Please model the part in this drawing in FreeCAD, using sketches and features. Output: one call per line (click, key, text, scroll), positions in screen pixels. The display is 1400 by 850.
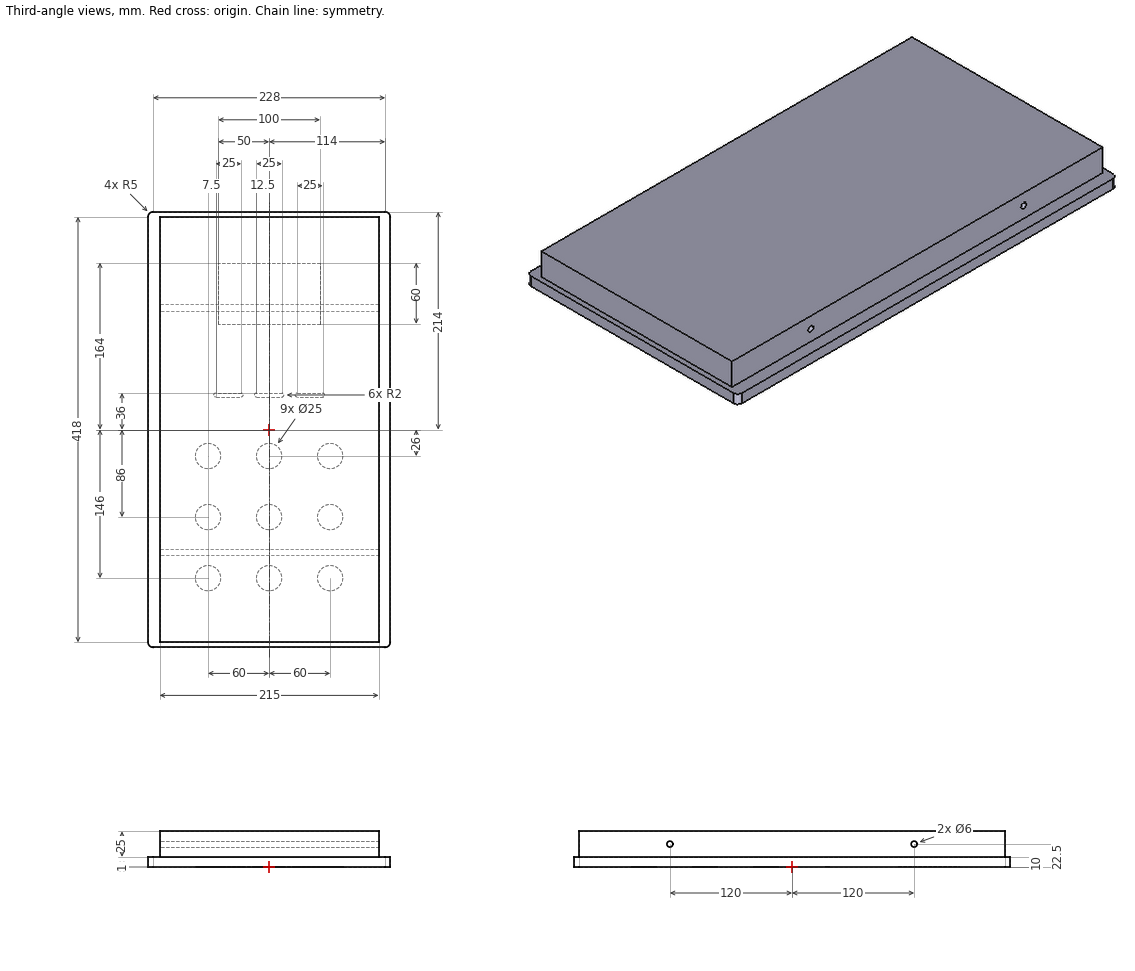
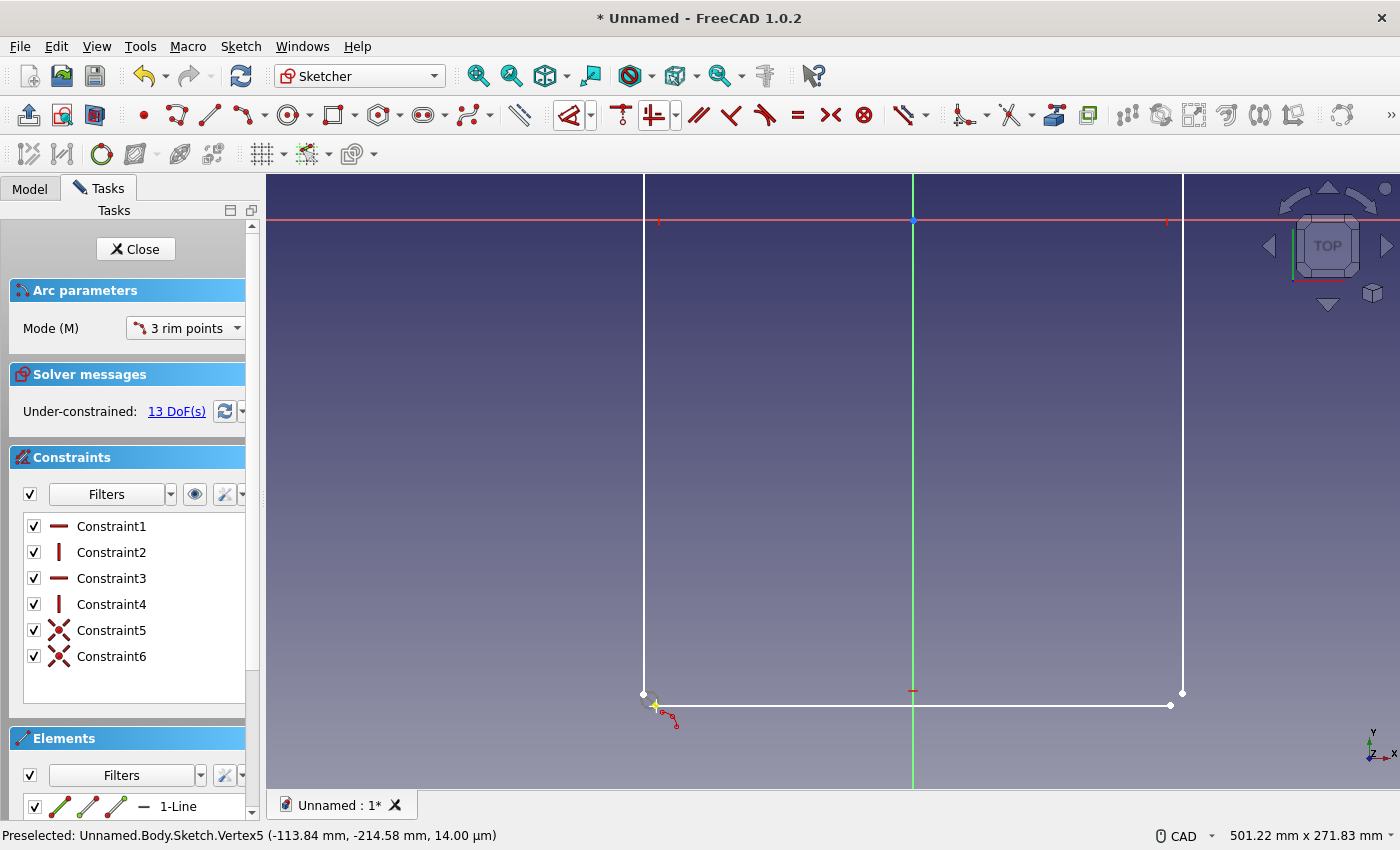
scroll(648, 701, up, 8)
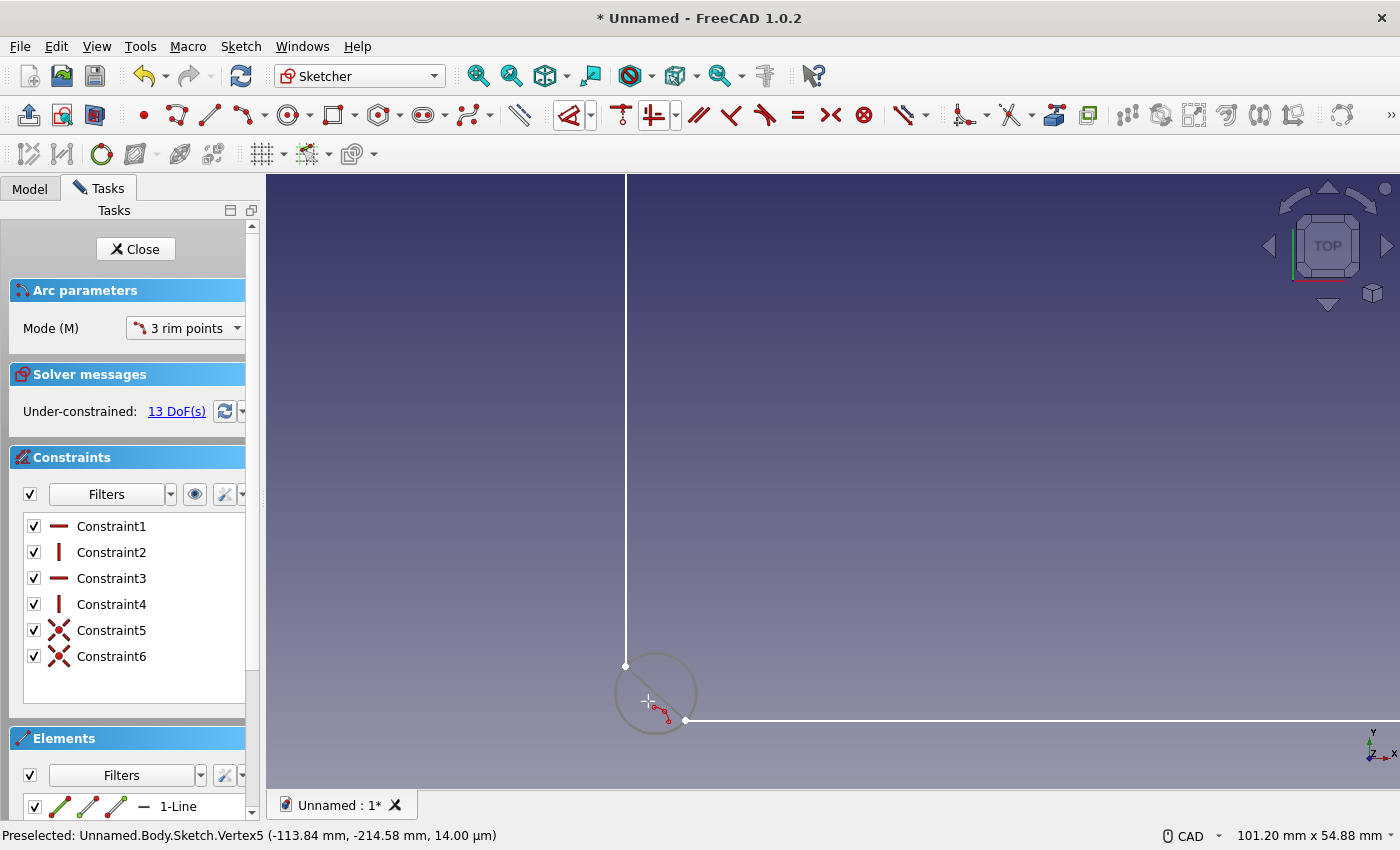
click(644, 698)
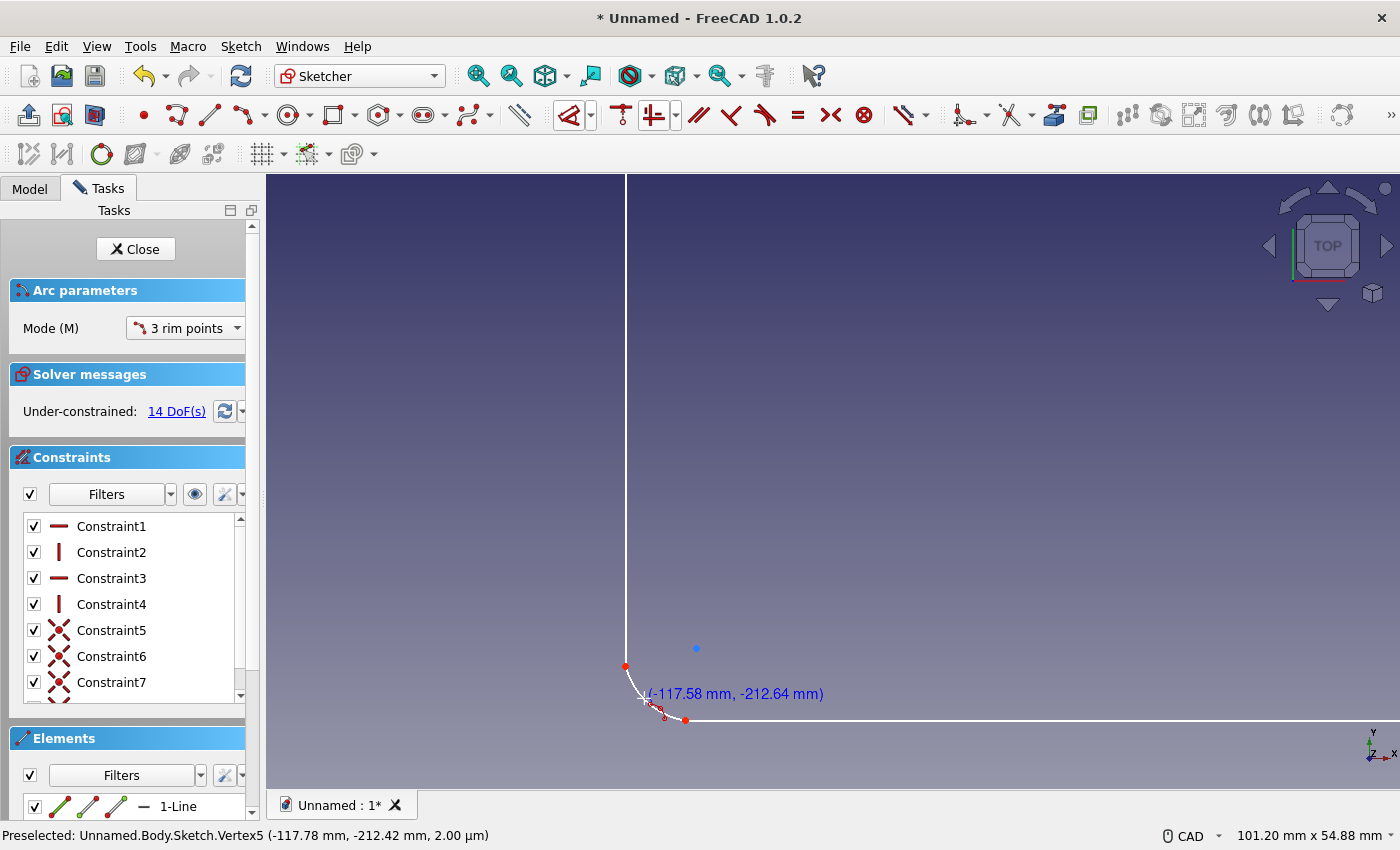
scroll(645, 698, down, 12)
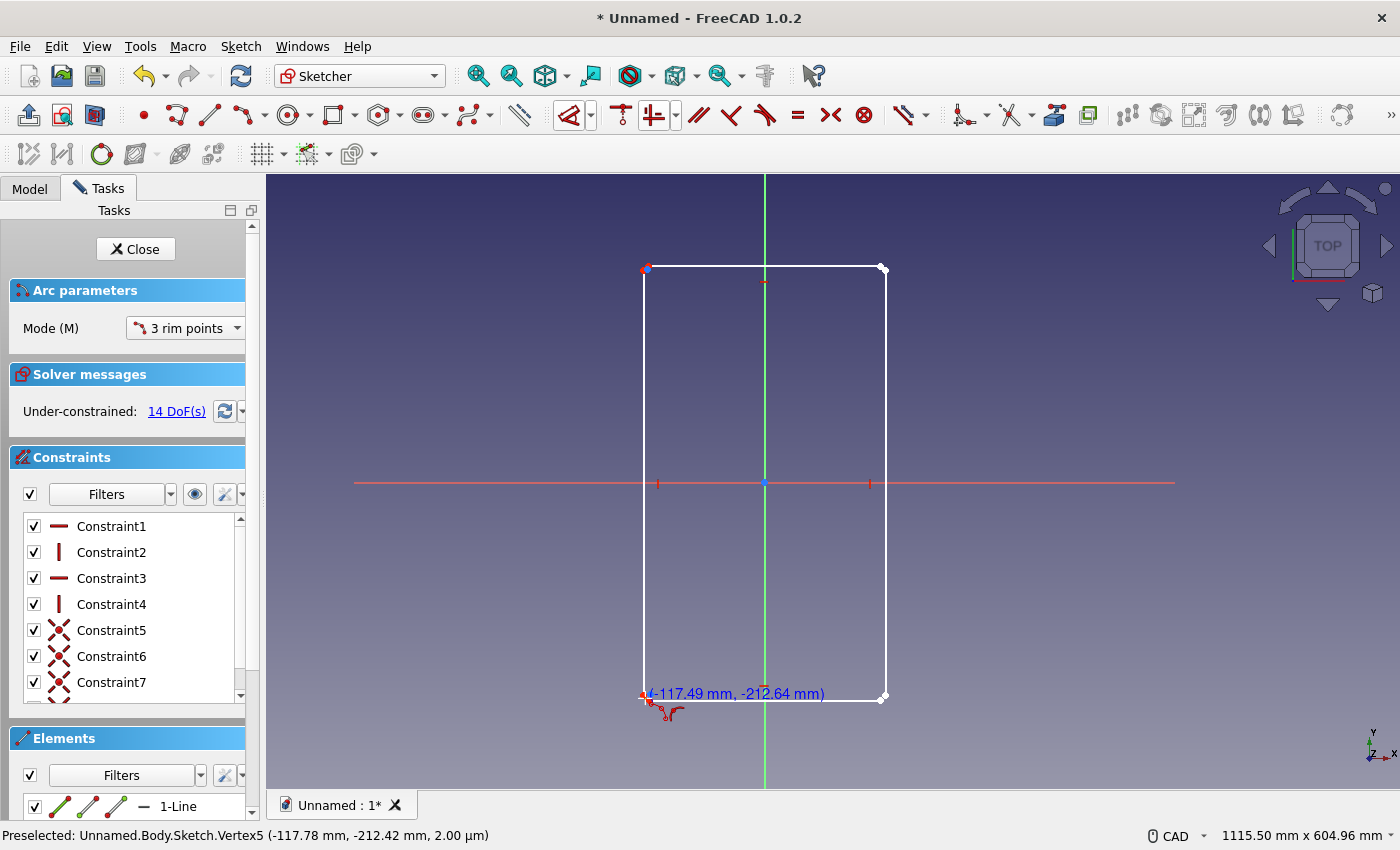
scroll(881, 700, up, 4)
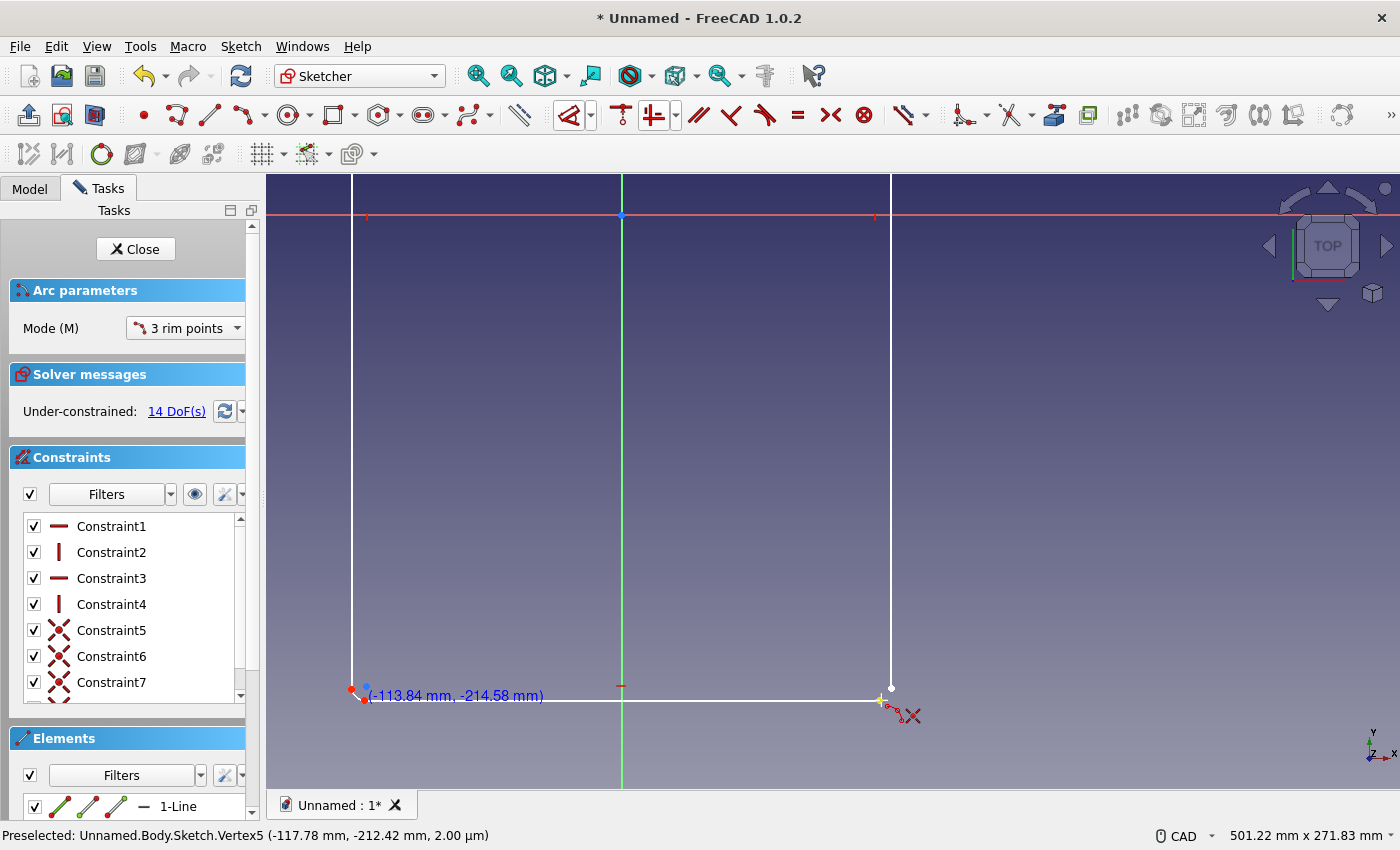
click(879, 701)
click(891, 689)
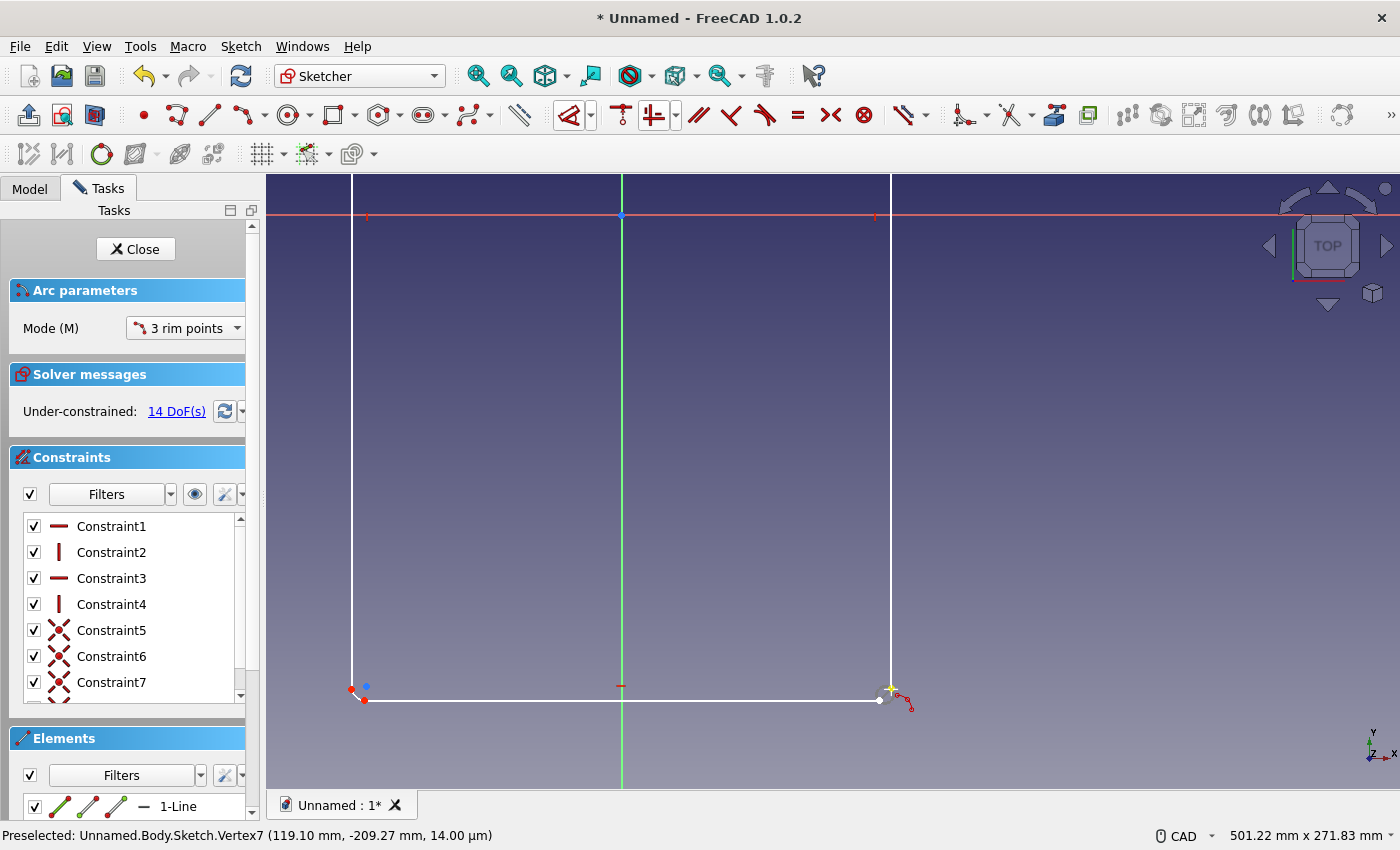
scroll(888, 696, up, 8)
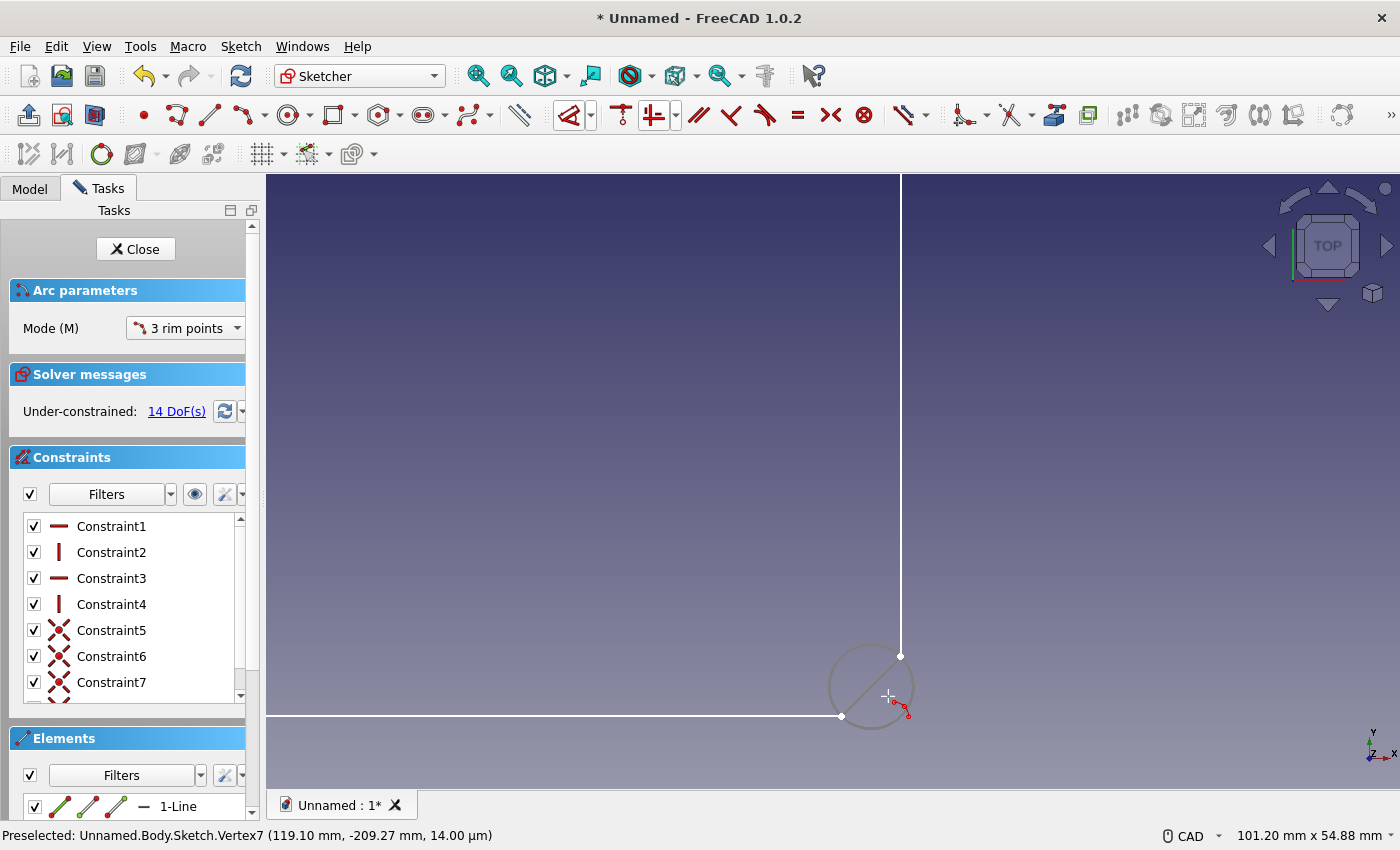
click(883, 694)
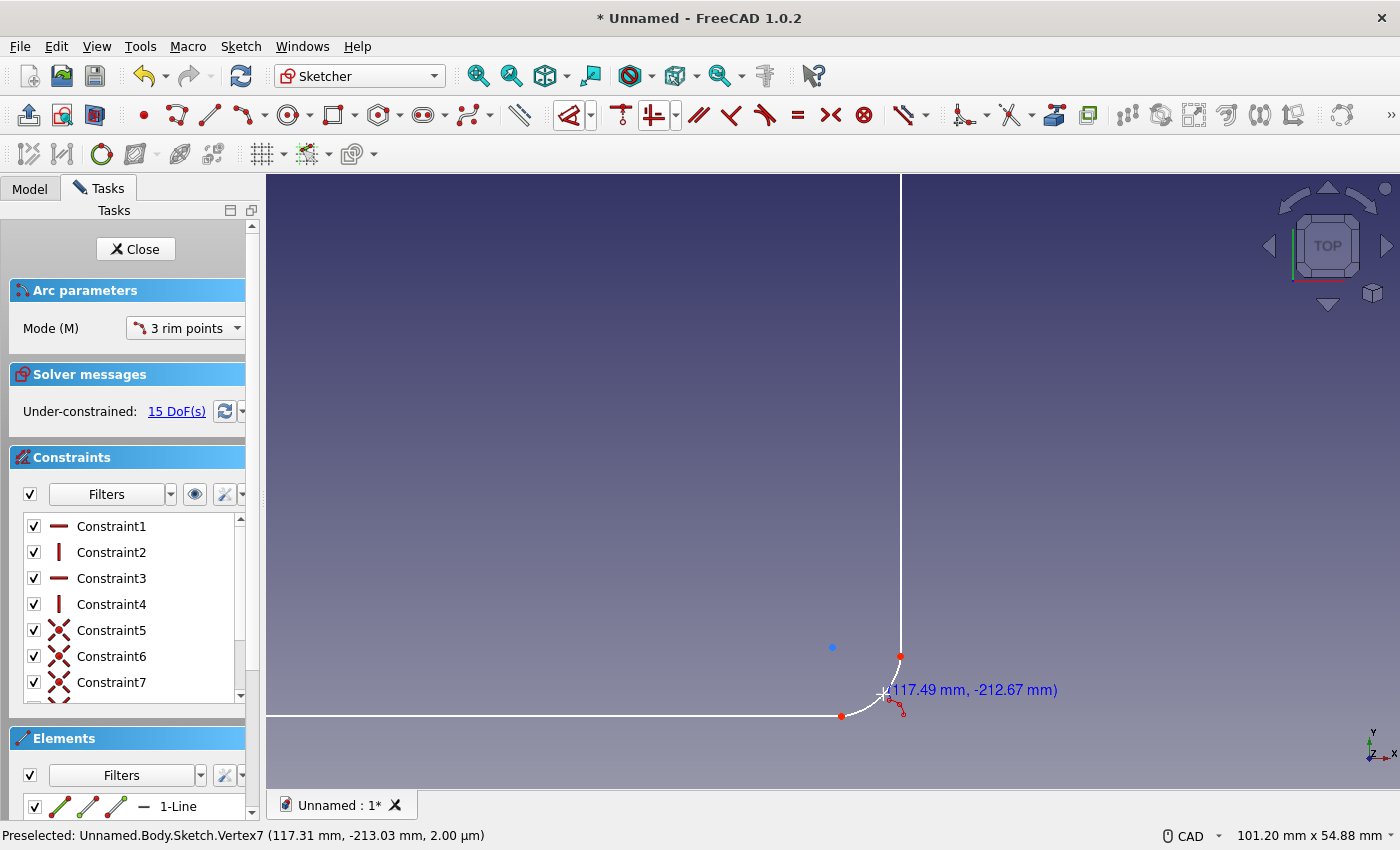
scroll(884, 698, down, 12)